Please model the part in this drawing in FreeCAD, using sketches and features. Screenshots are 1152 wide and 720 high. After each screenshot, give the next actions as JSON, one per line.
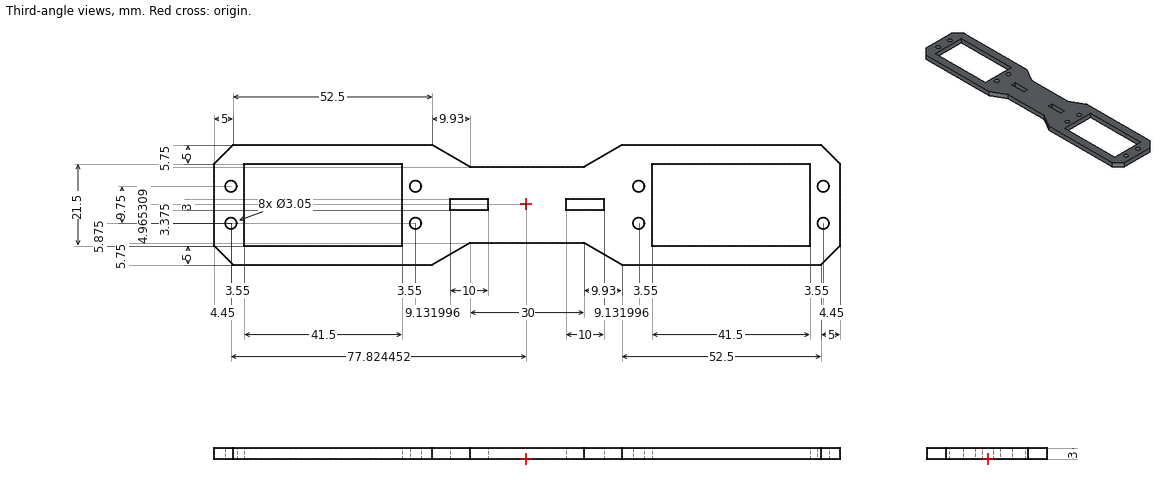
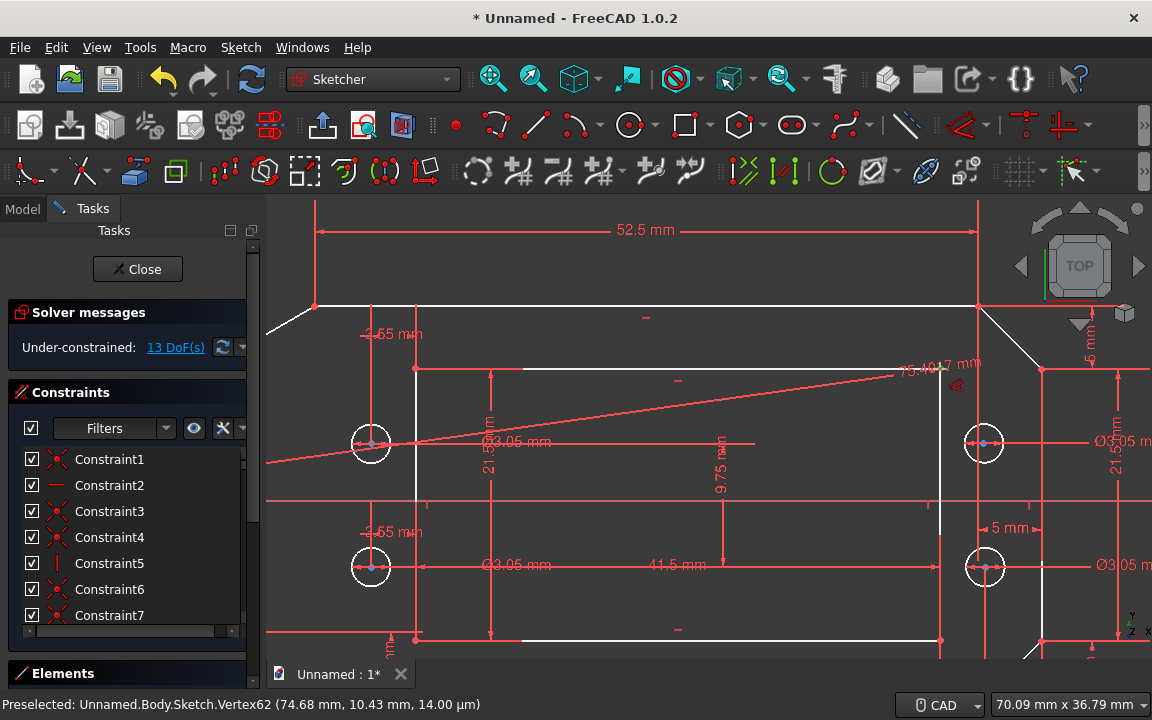
{"action": "left_click", "coordinate": [984, 443]}
{"action": "left_click", "coordinate": [962, 335]}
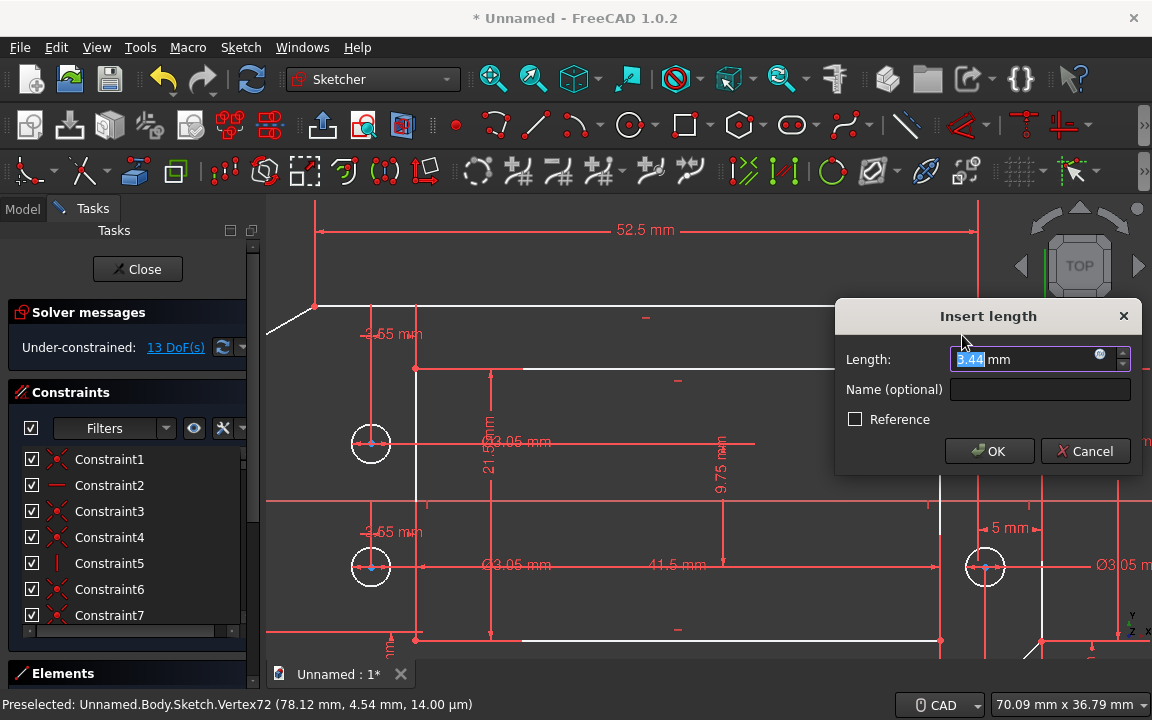
{"action": "type", "text": "3.55"}
{"action": "key", "text": "Return"}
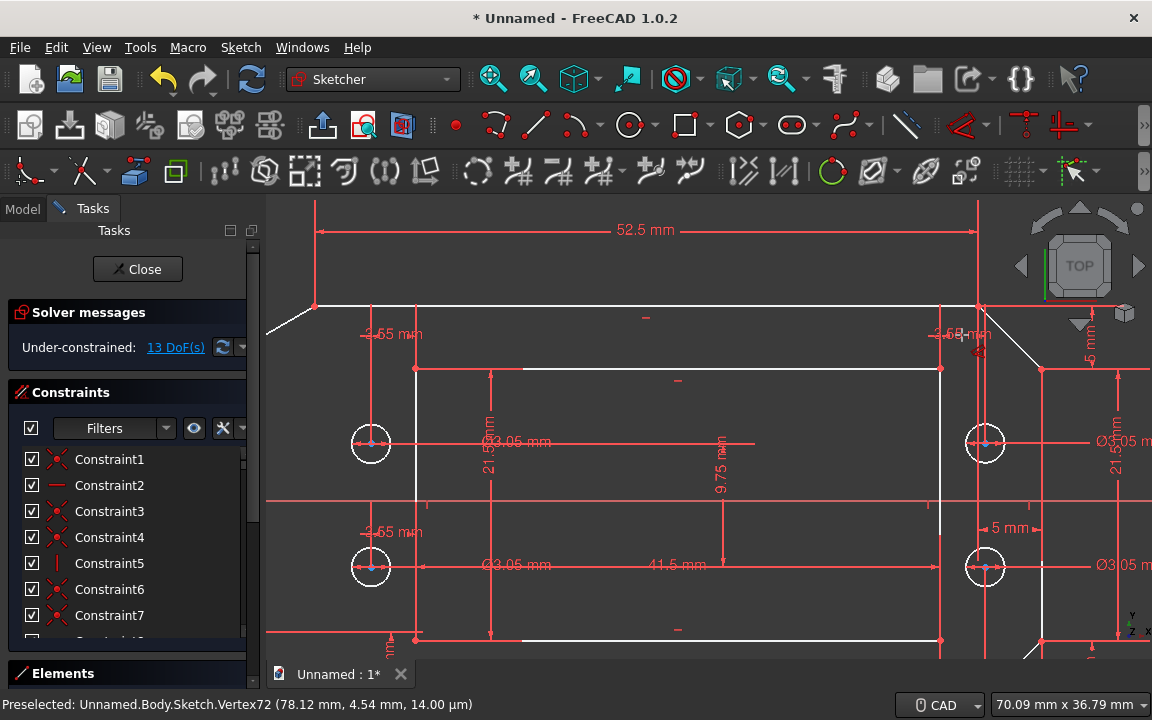
{"action": "scroll", "coordinate": [851, 402], "scroll_direction": "down", "scroll_amount": 7}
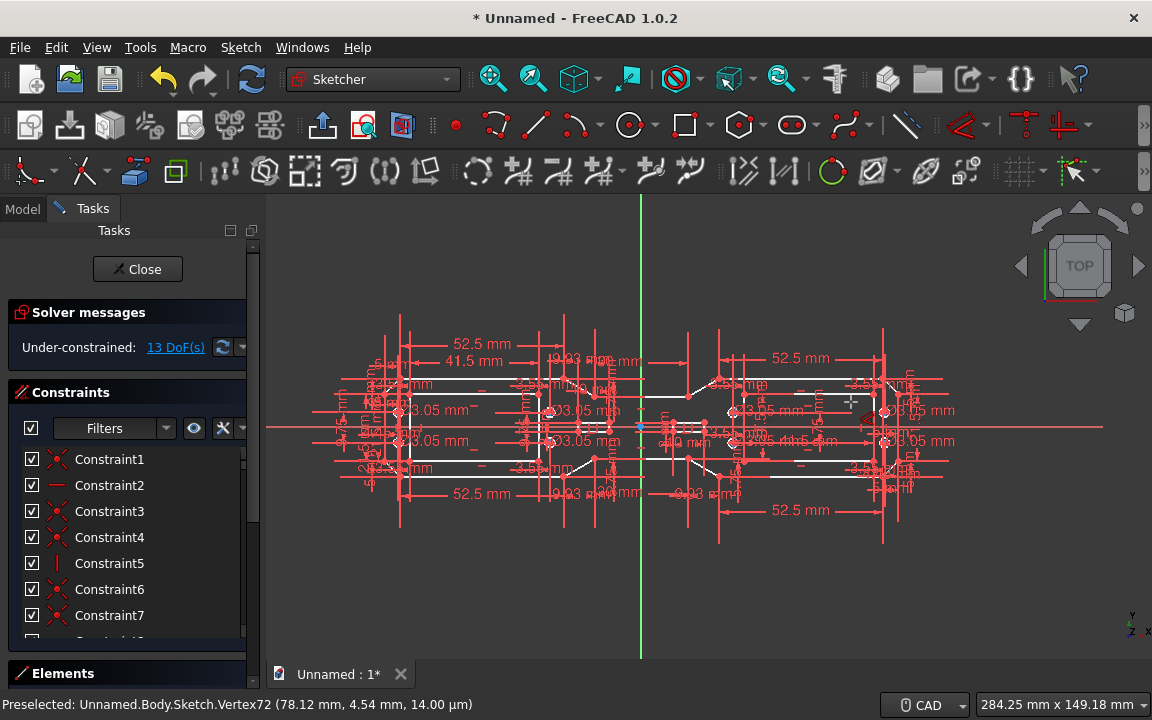
{"action": "scroll", "coordinate": [885, 443], "scroll_direction": "up", "scroll_amount": 2}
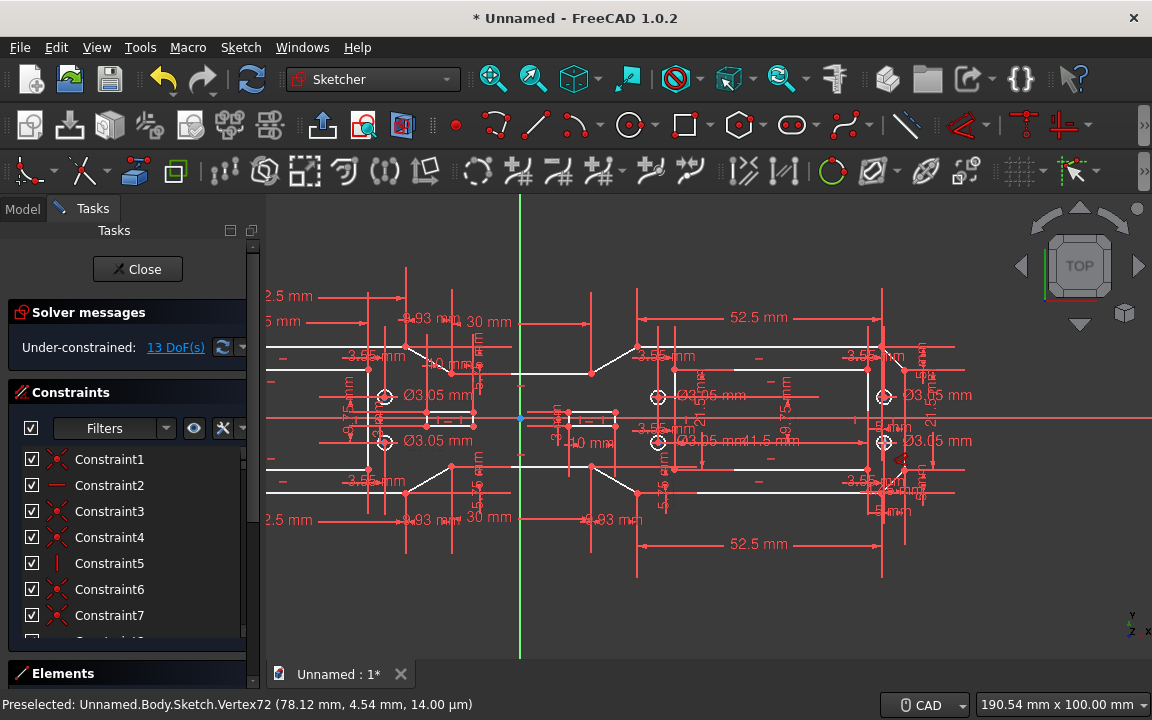
{"action": "left_click", "coordinate": [884, 443]}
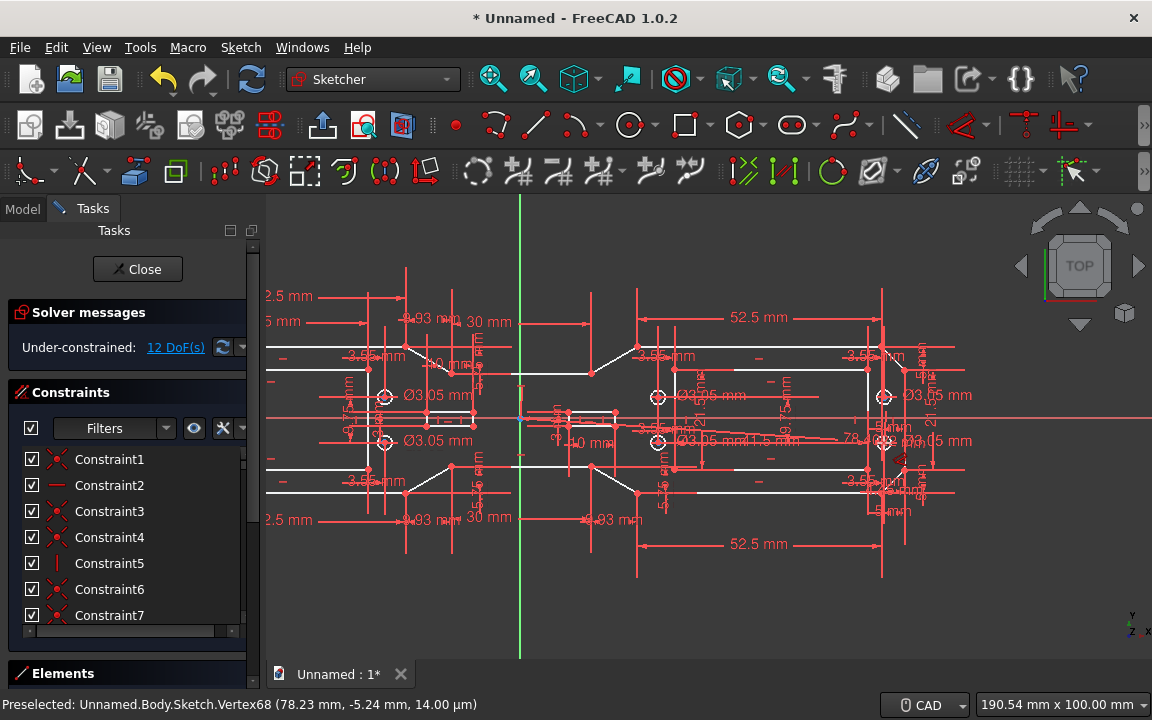
{"action": "left_click", "coordinate": [884, 397]}
{"action": "left_click", "coordinate": [966, 436]}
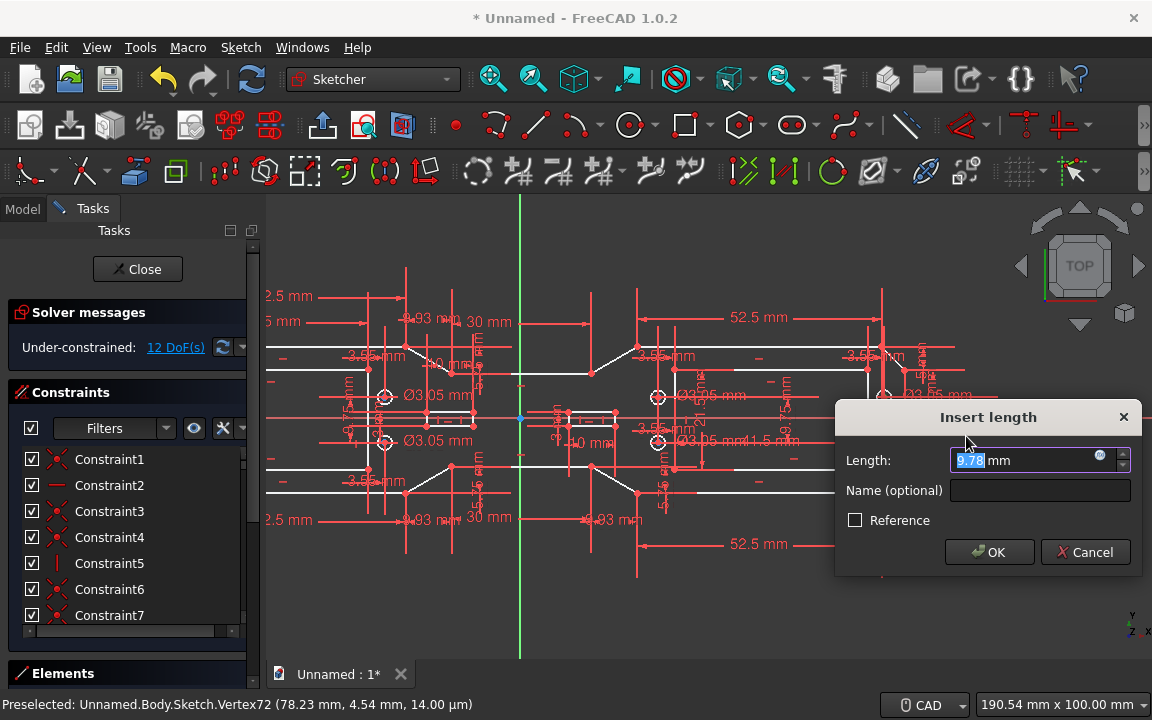
{"action": "type", "text": "9.75"}
{"action": "key", "text": "Return"}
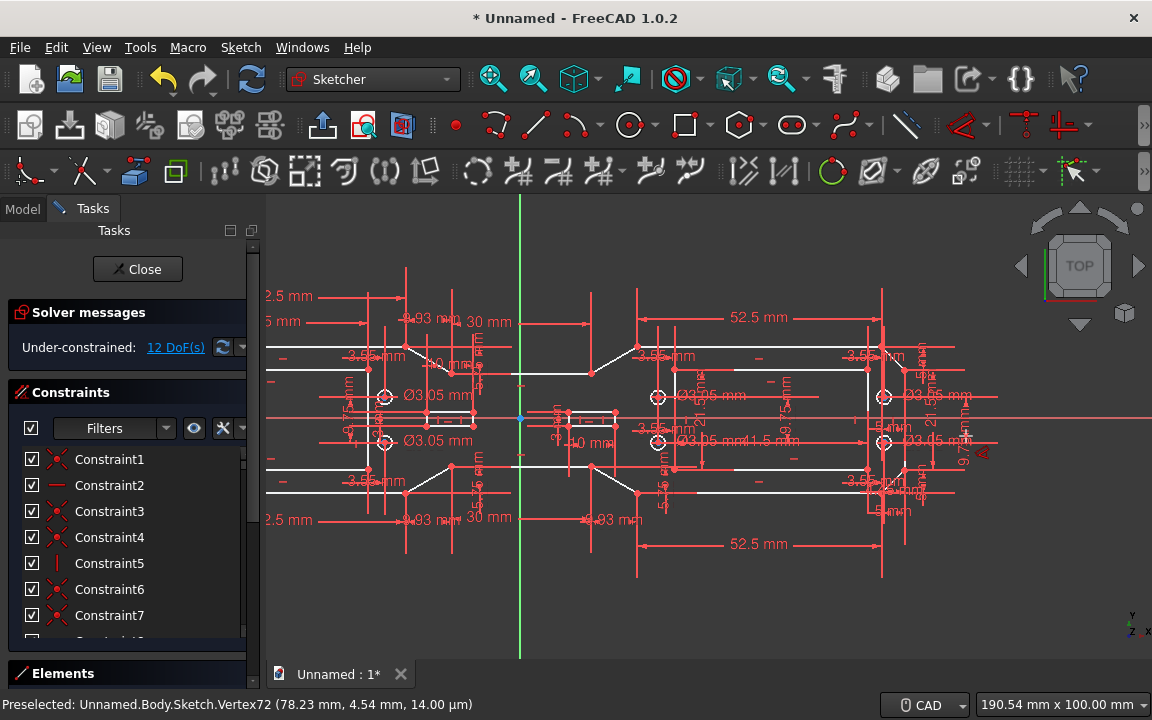
{"action": "scroll", "coordinate": [883, 442], "scroll_direction": "down", "scroll_amount": 2}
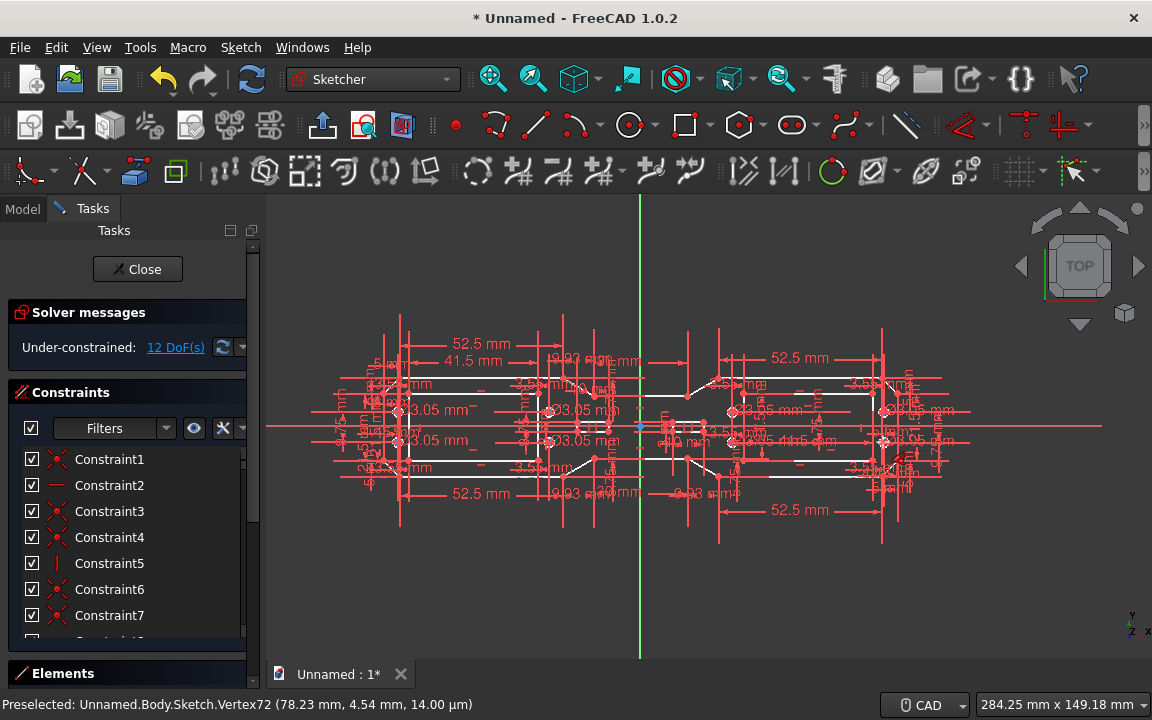
{"action": "scroll", "coordinate": [409, 461], "scroll_direction": "up", "scroll_amount": 4}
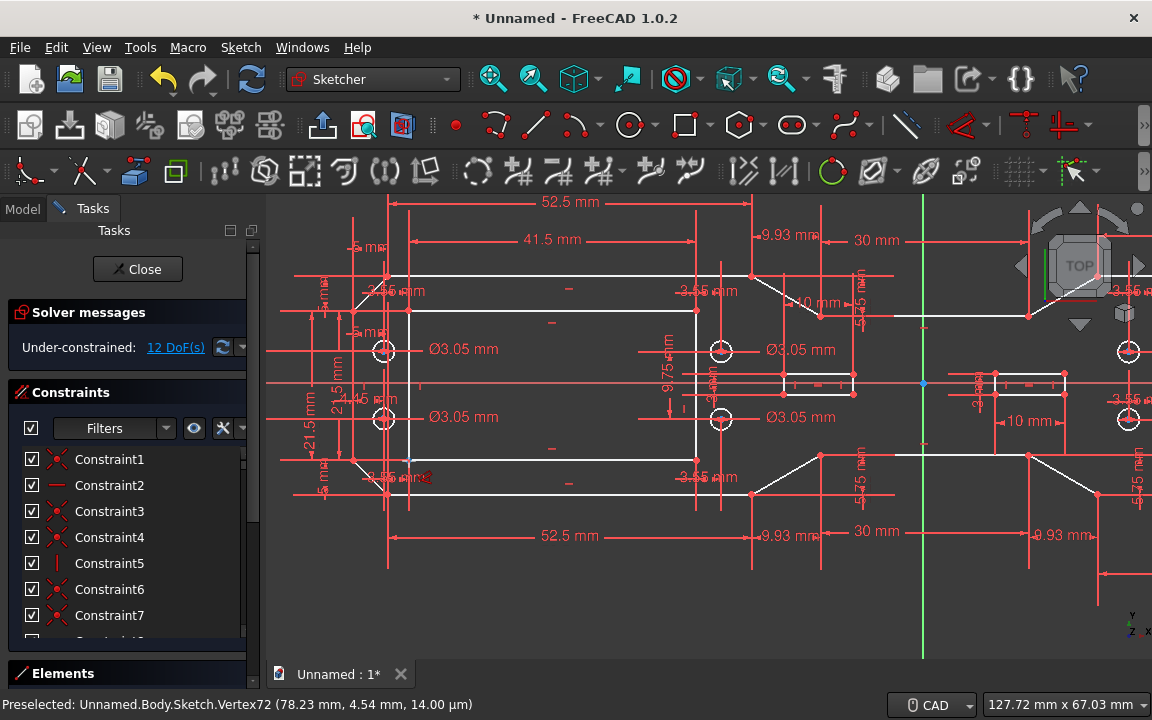
{"action": "left_click", "coordinate": [409, 460]}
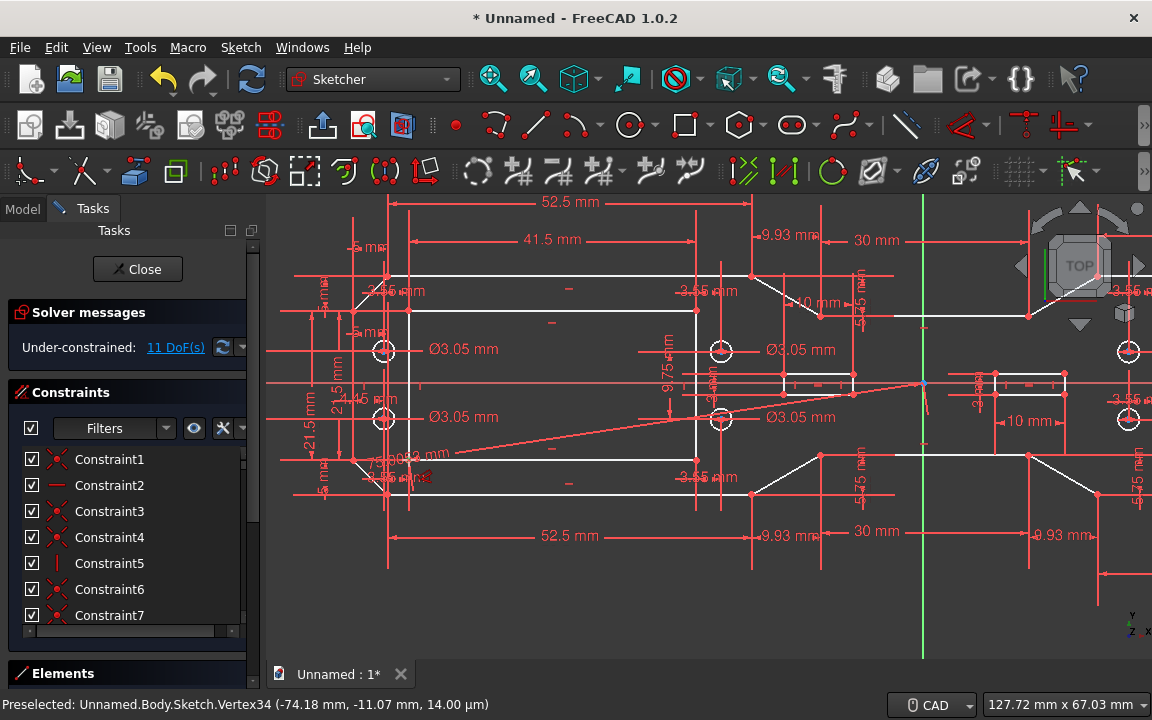
{"action": "left_click", "coordinate": [384, 419]}
{"action": "left_click", "coordinate": [443, 439]}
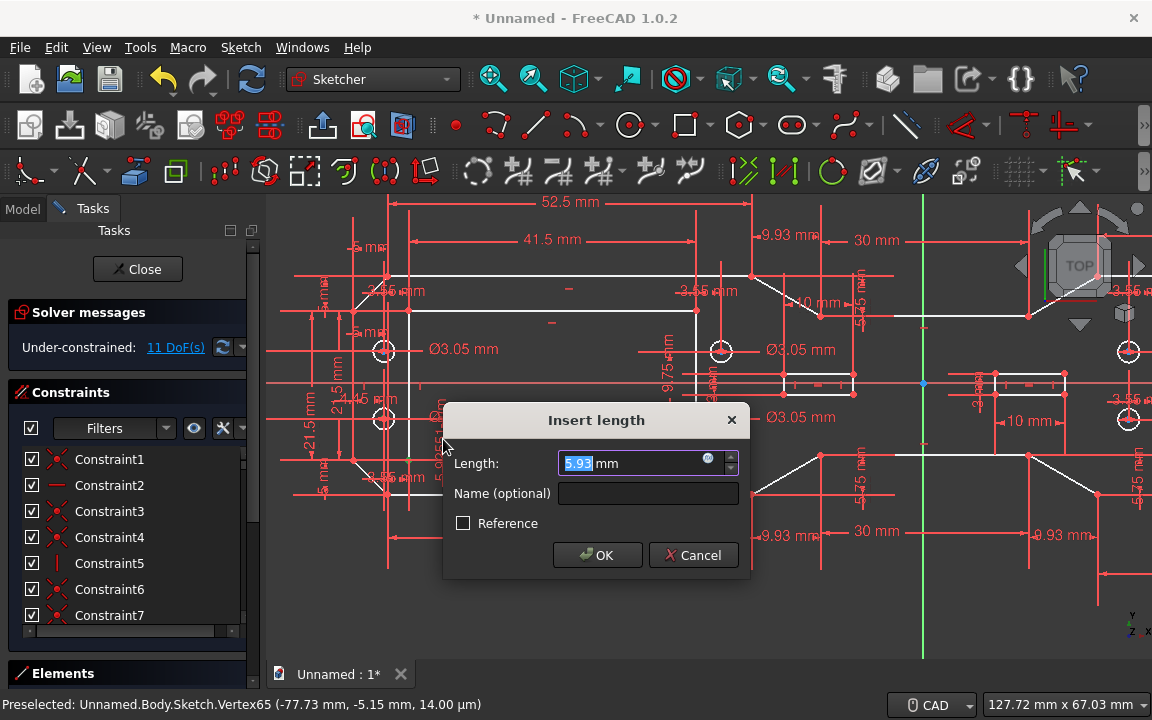
{"action": "type", "text": "5.875"}
{"action": "key", "text": "Return"}